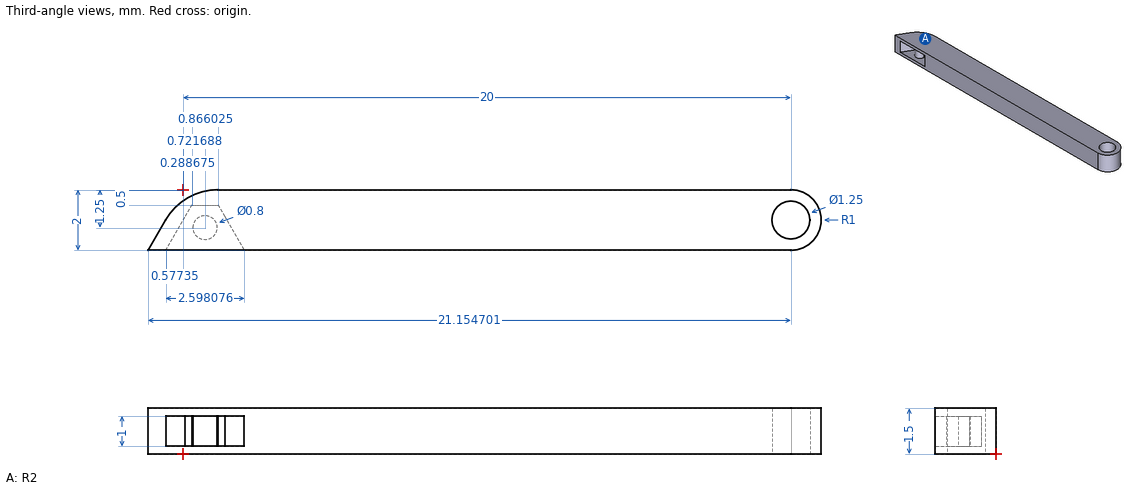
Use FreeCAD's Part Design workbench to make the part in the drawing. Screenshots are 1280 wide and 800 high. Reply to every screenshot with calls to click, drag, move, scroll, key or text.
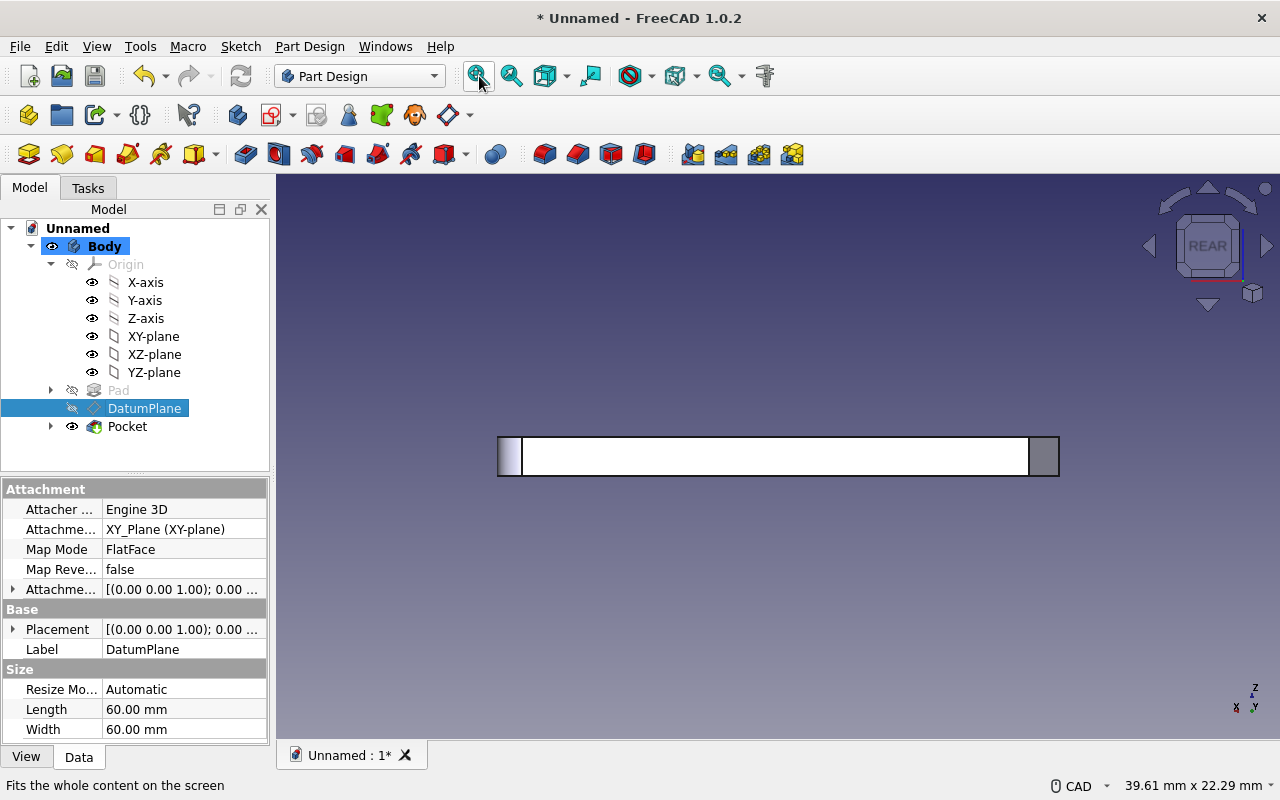
click(1029, 455)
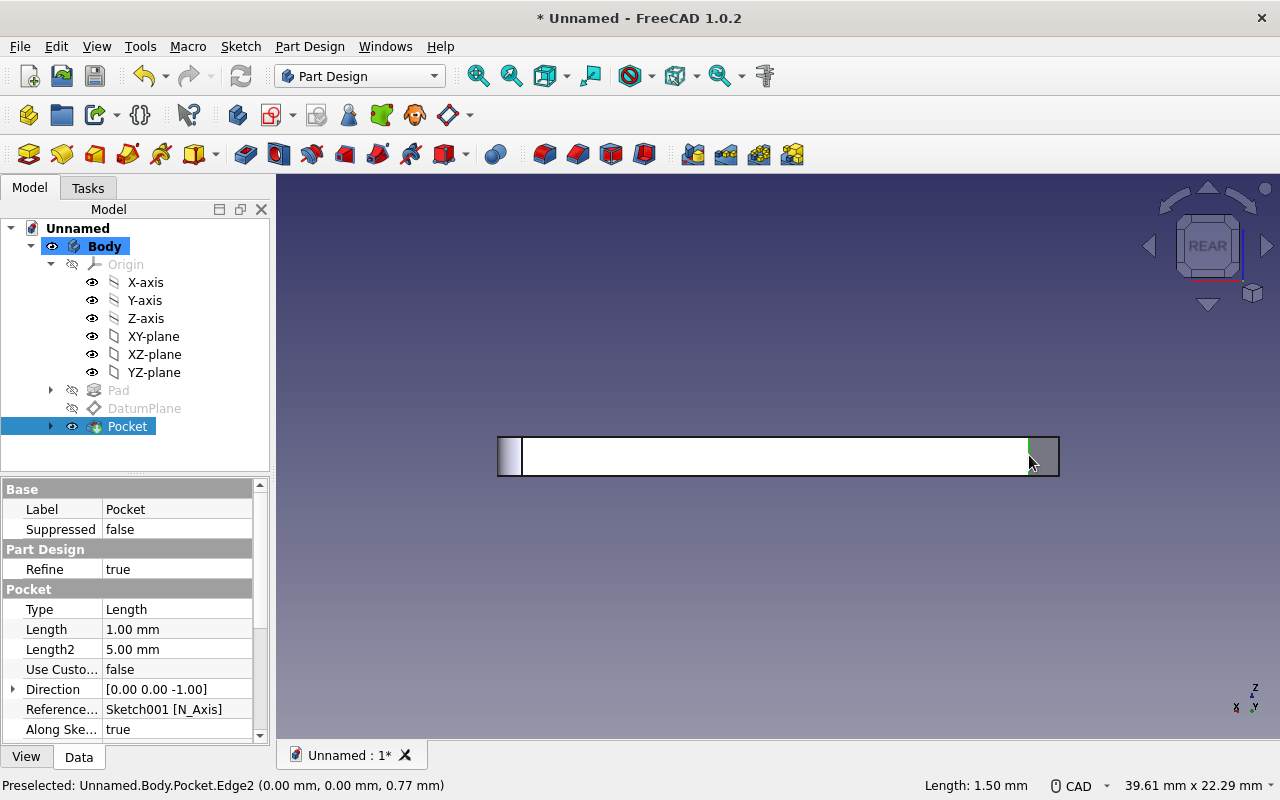
click(545, 154)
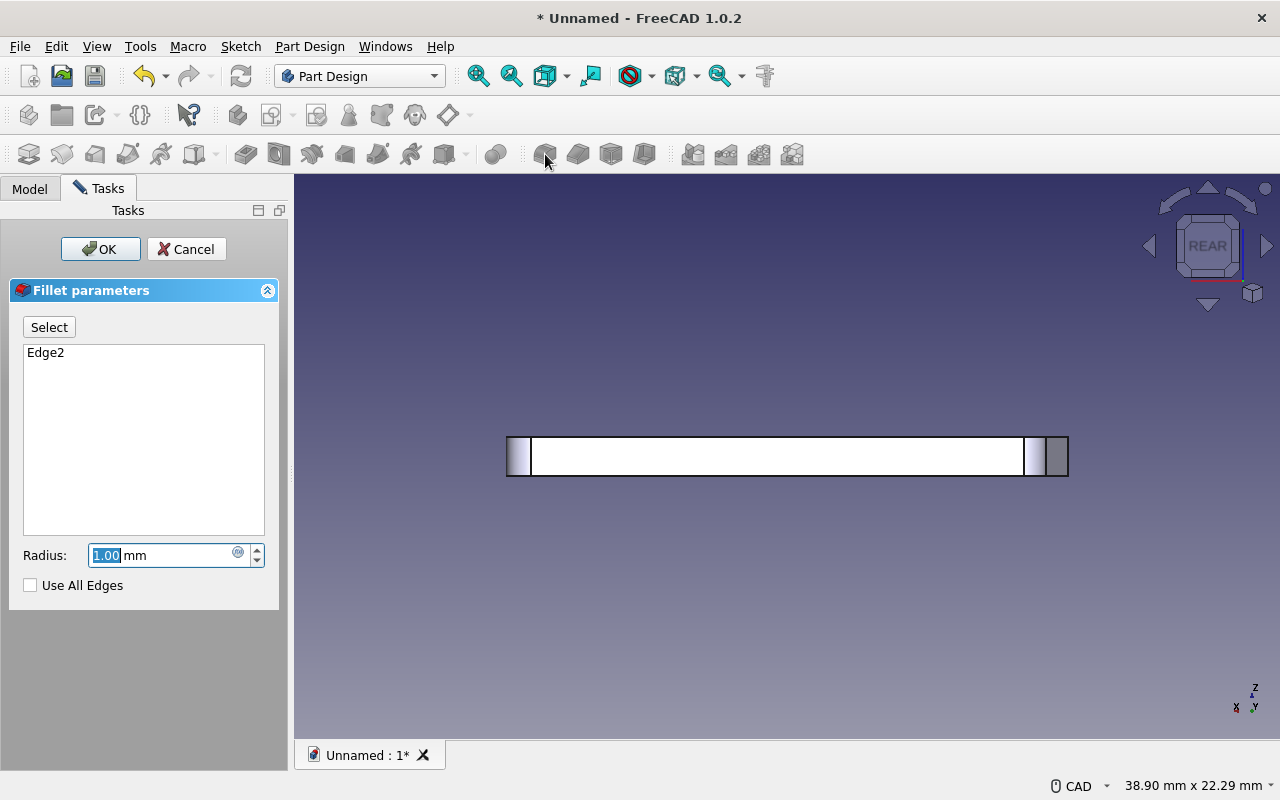
text(2)
key(Tab)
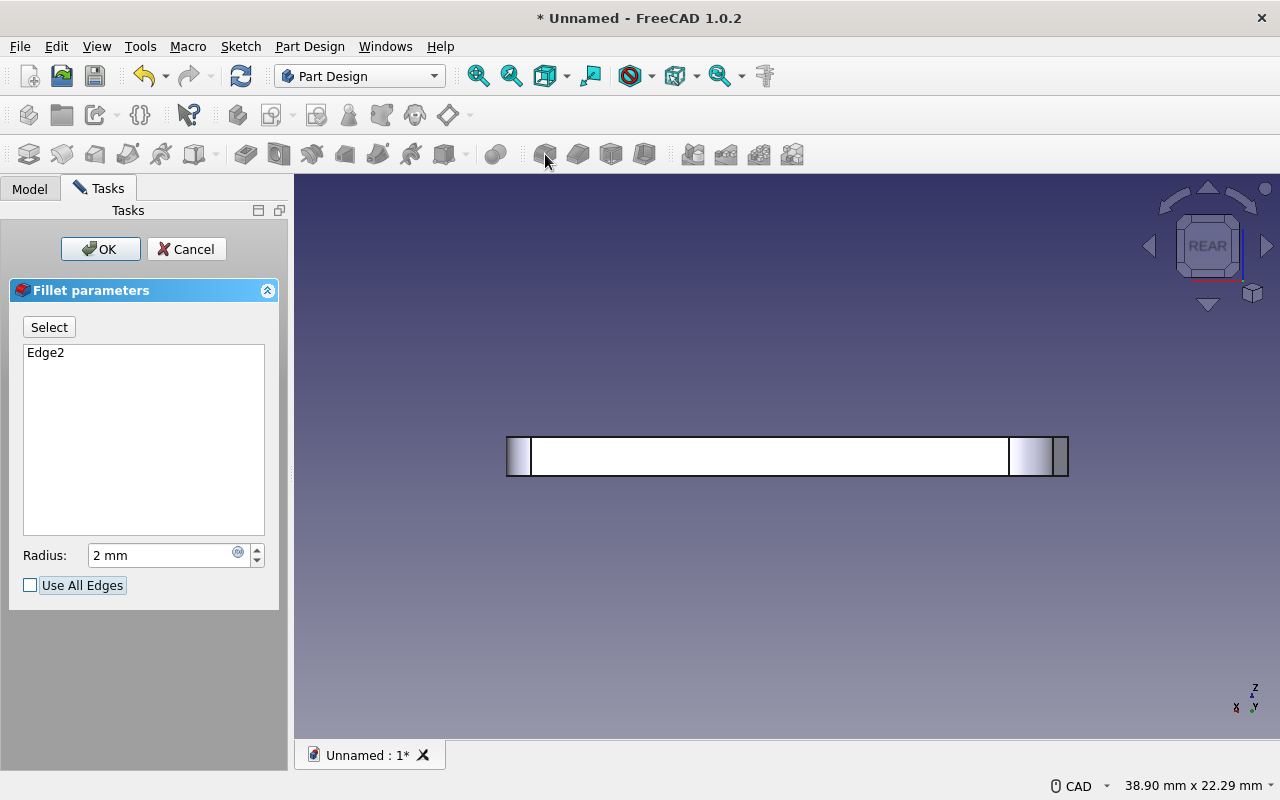
click(101, 249)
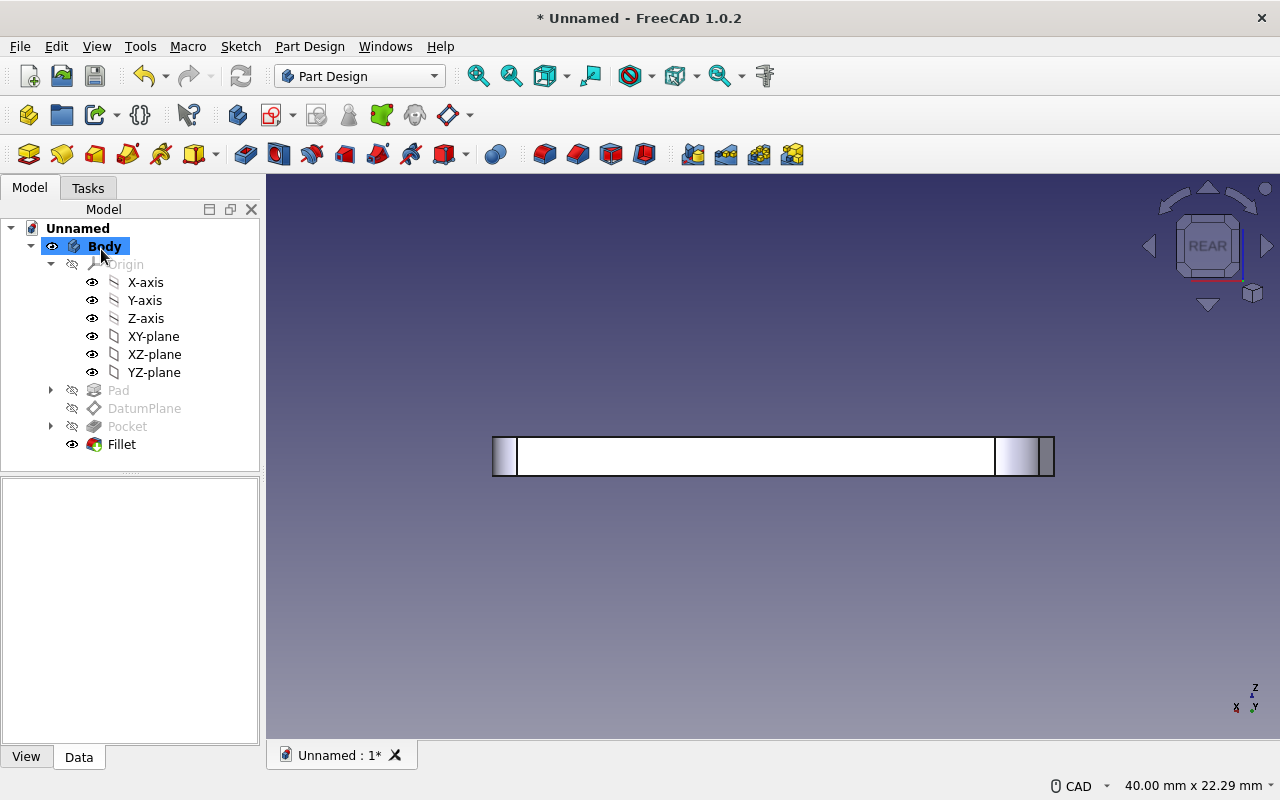
key(0)